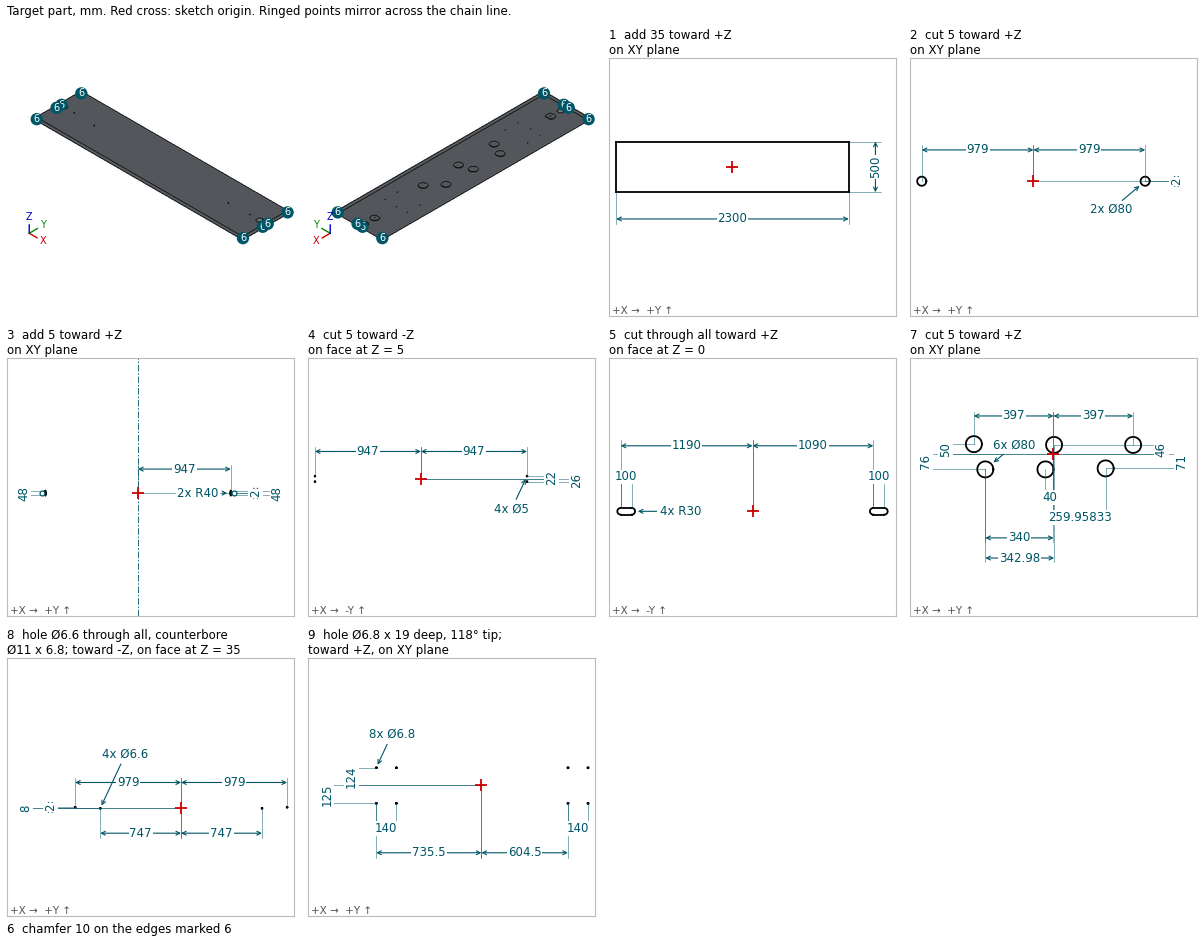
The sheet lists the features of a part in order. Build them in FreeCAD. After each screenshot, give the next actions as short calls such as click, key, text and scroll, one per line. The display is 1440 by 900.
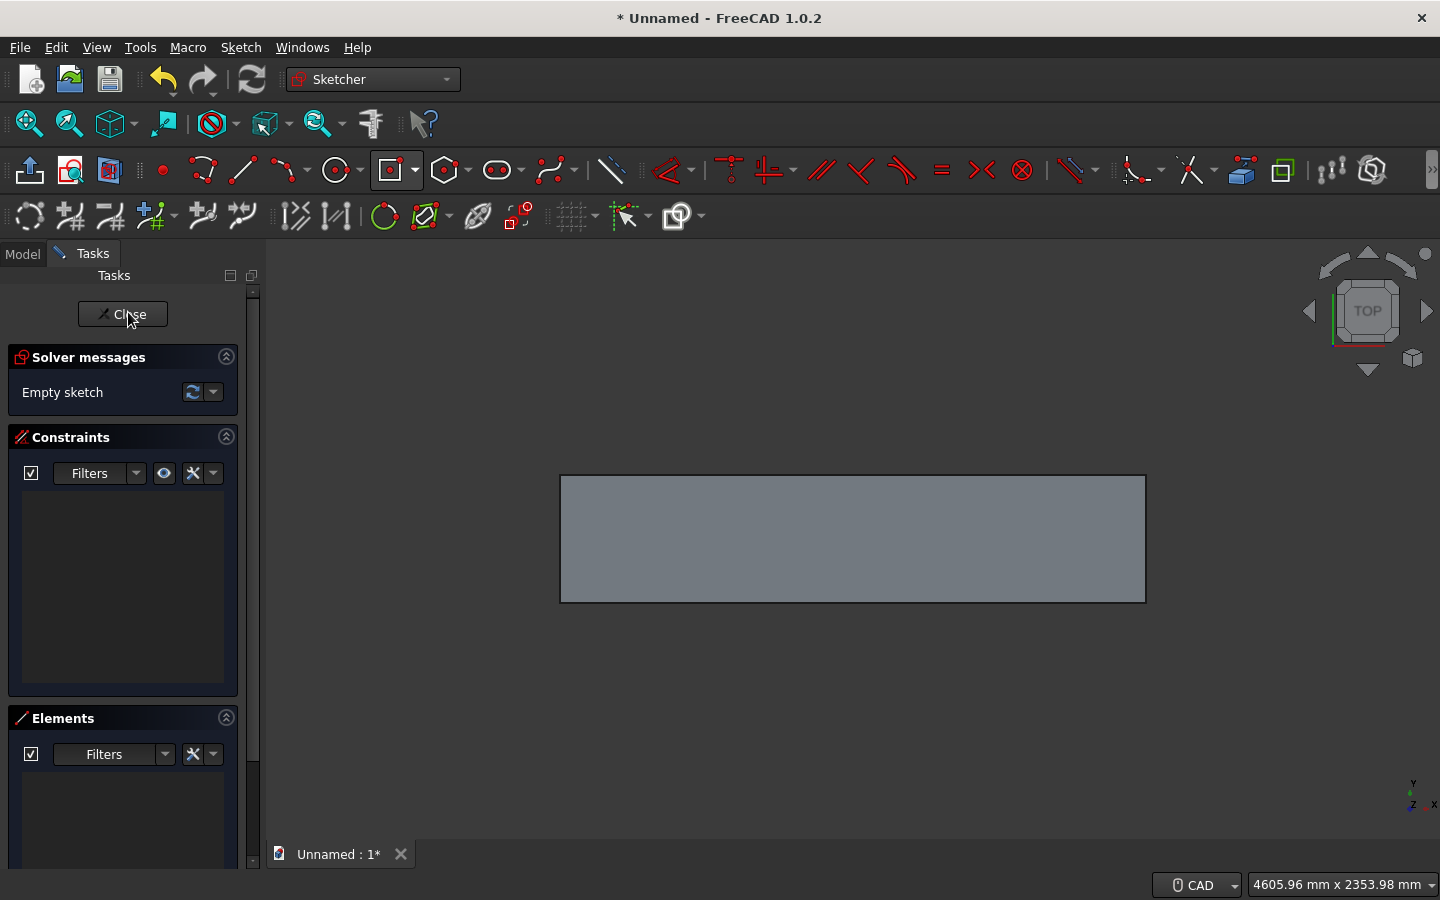
key(q)
key(s)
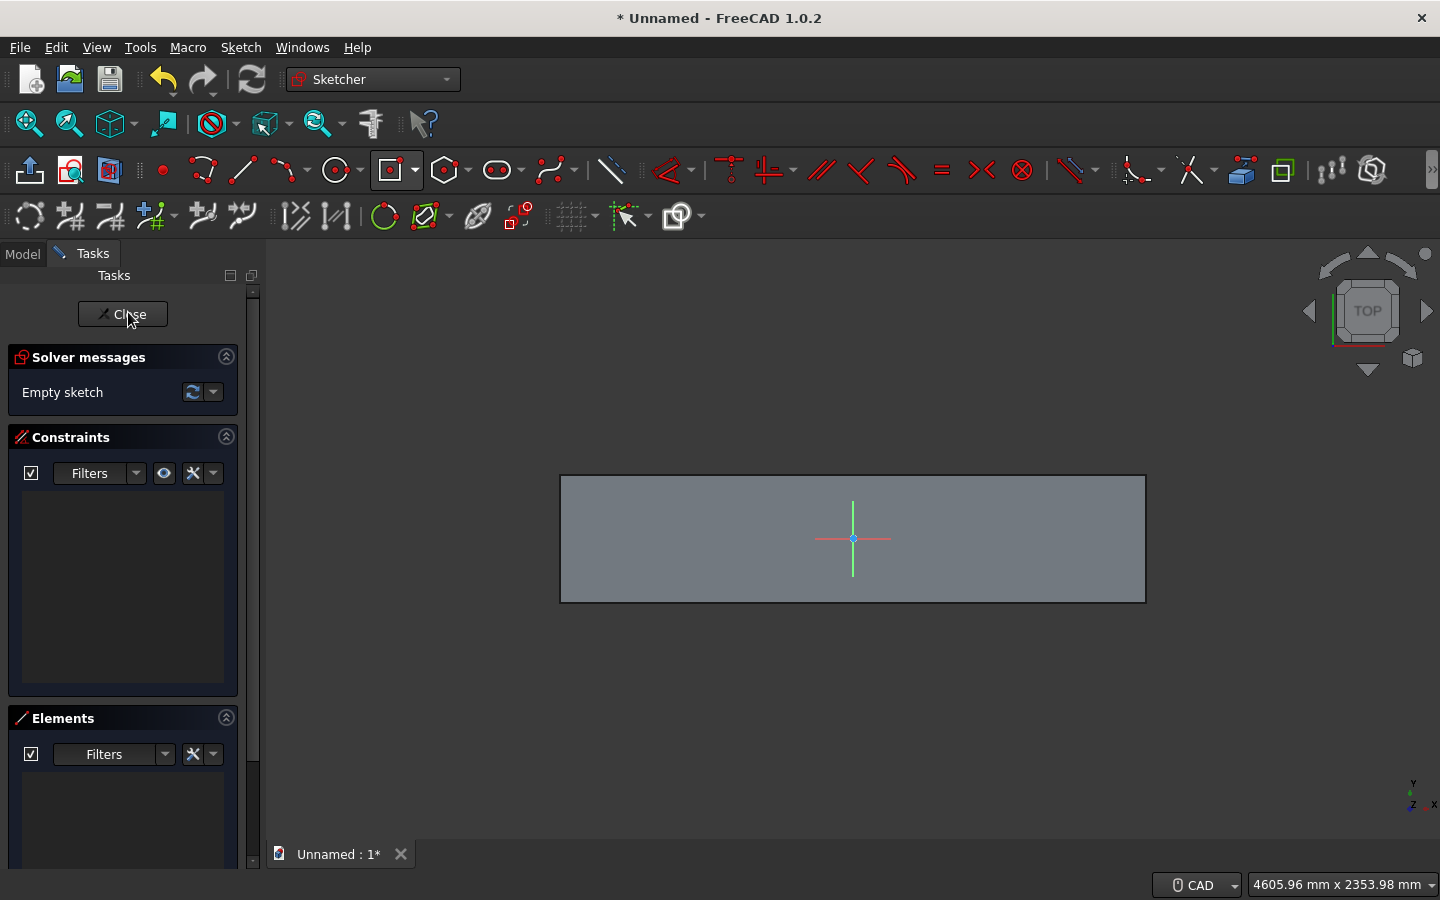
click(336, 170)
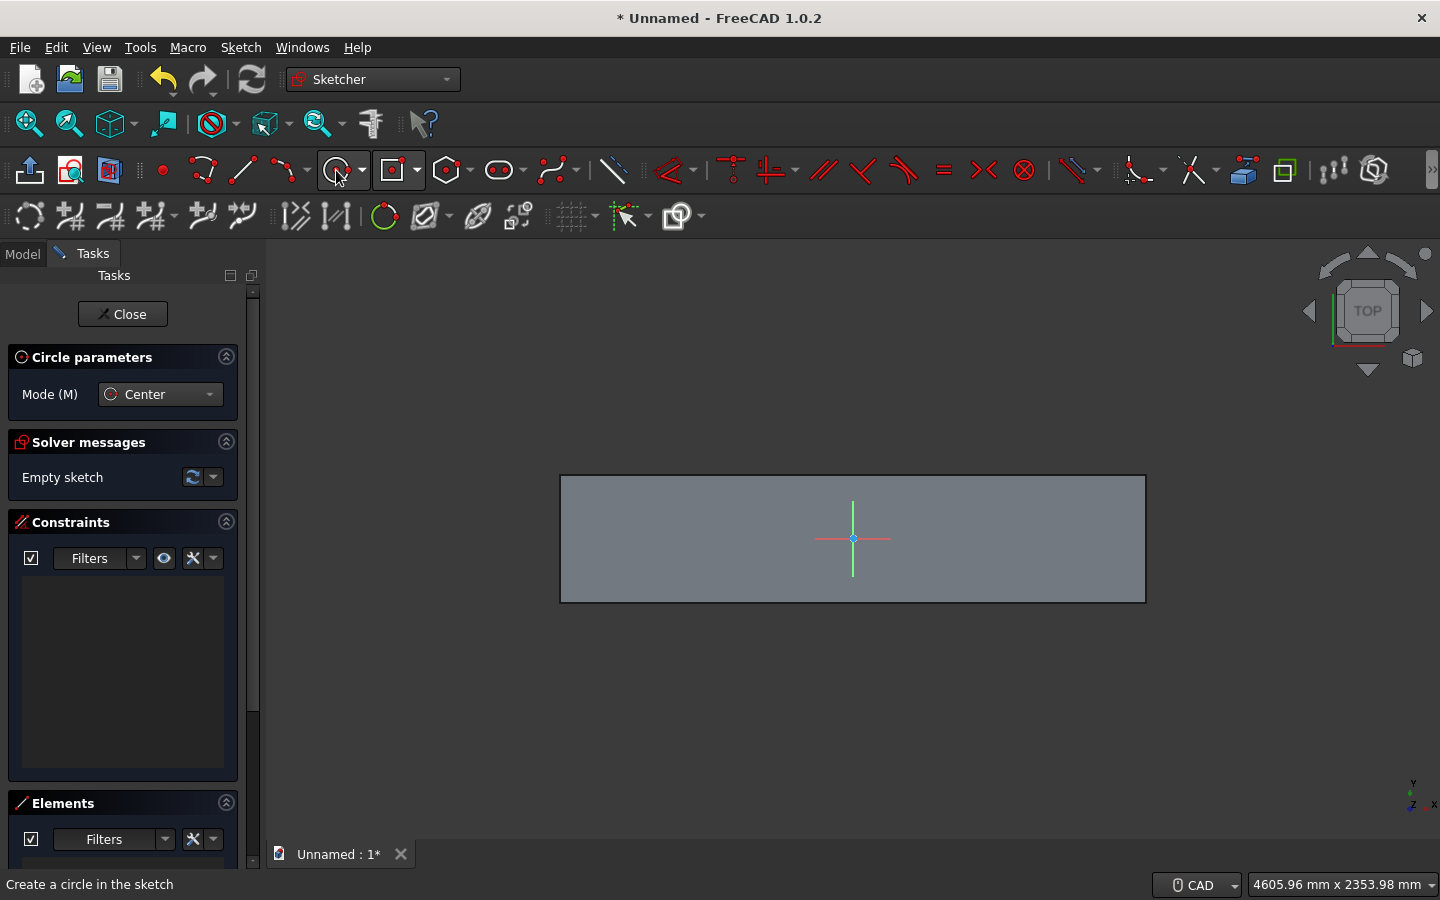
scroll(1103, 538, up, 18)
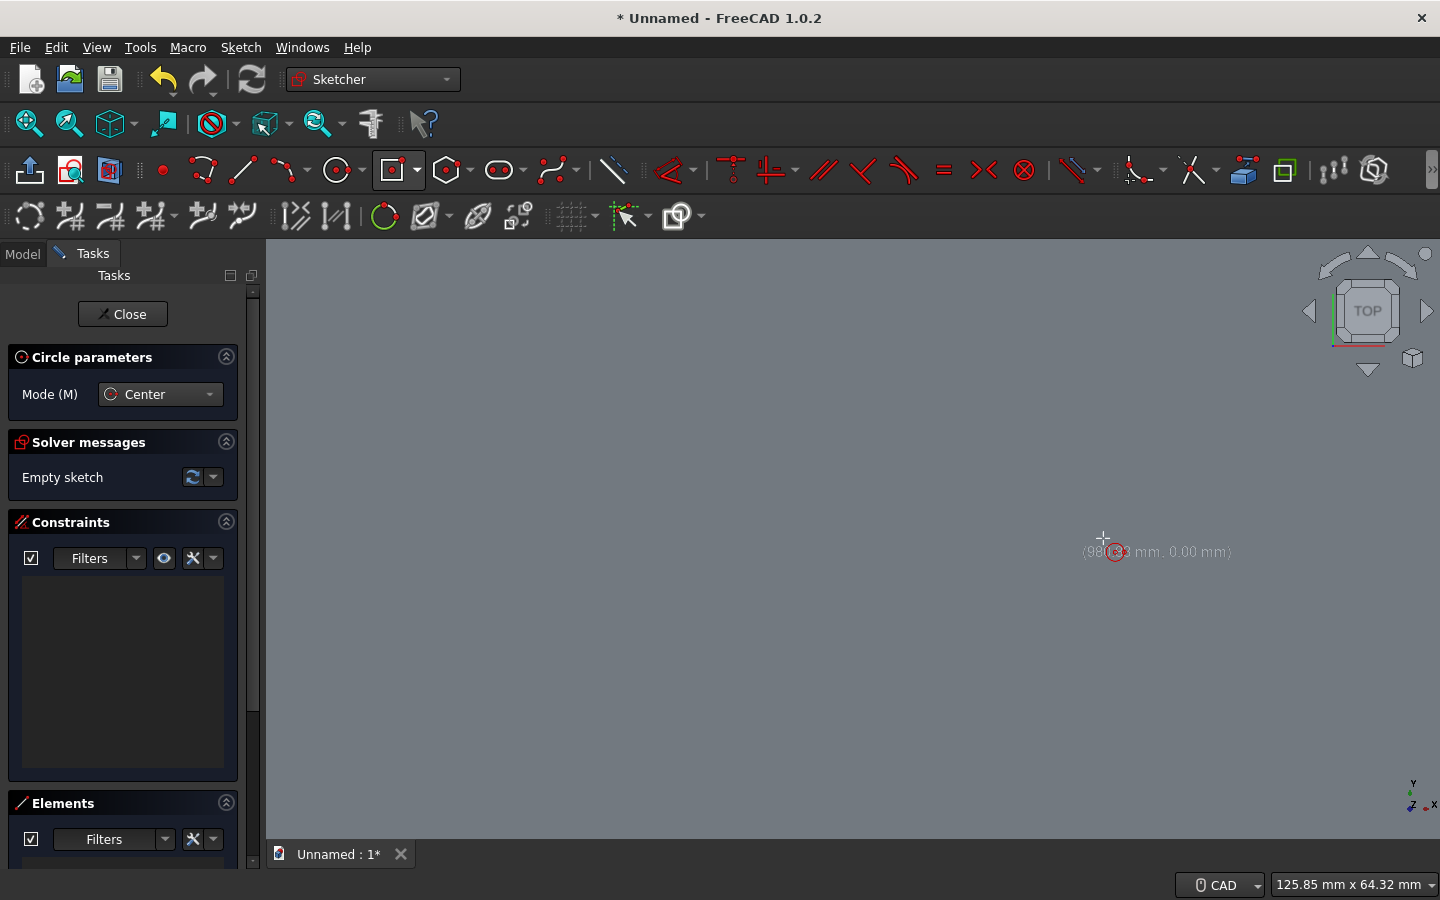
click(1061, 538)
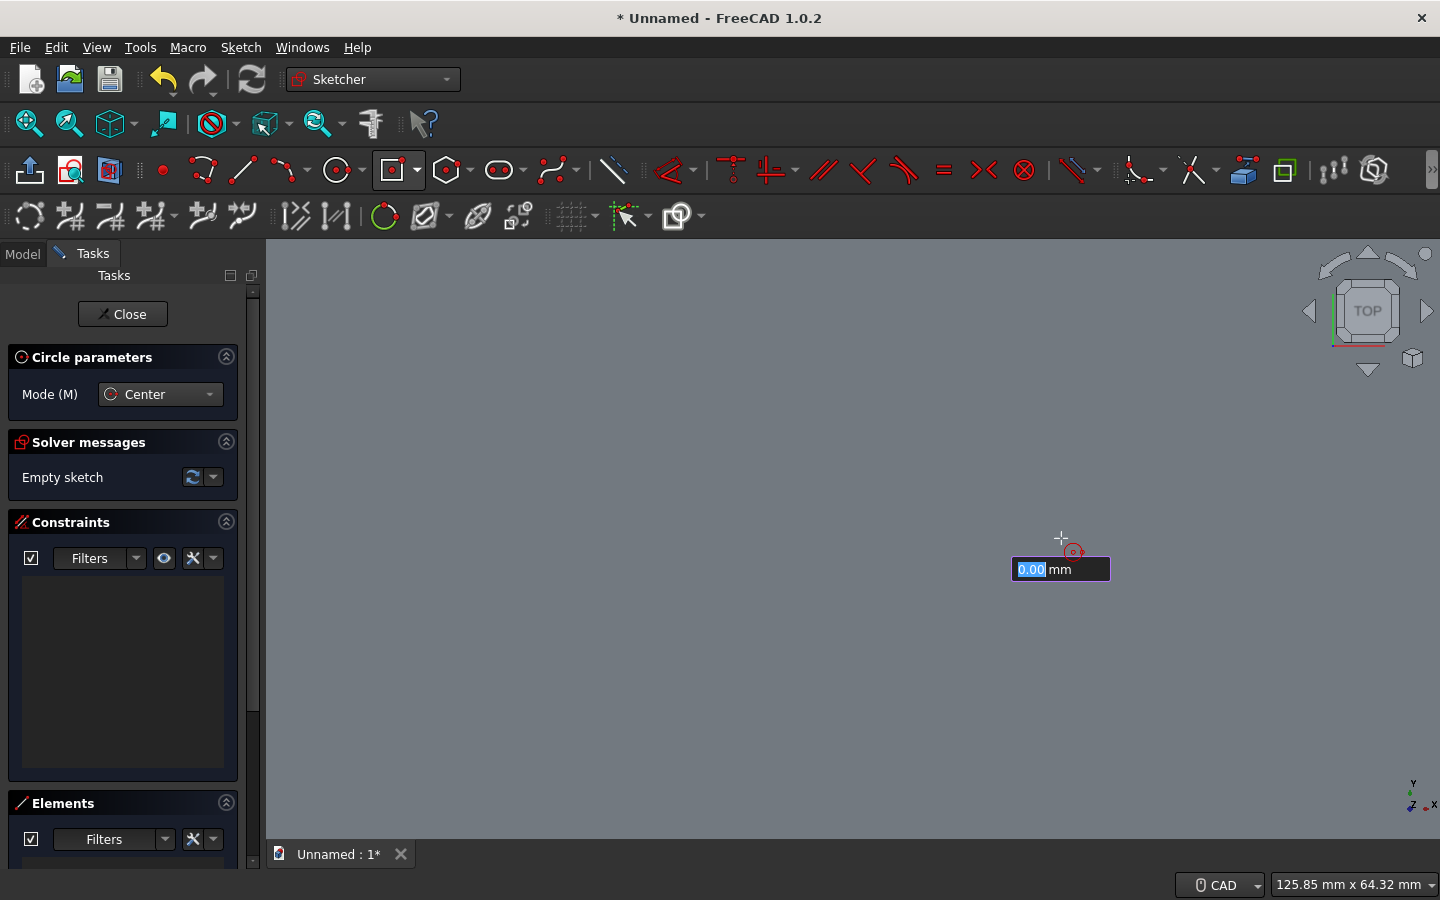
scroll(1161, 539, down, 16)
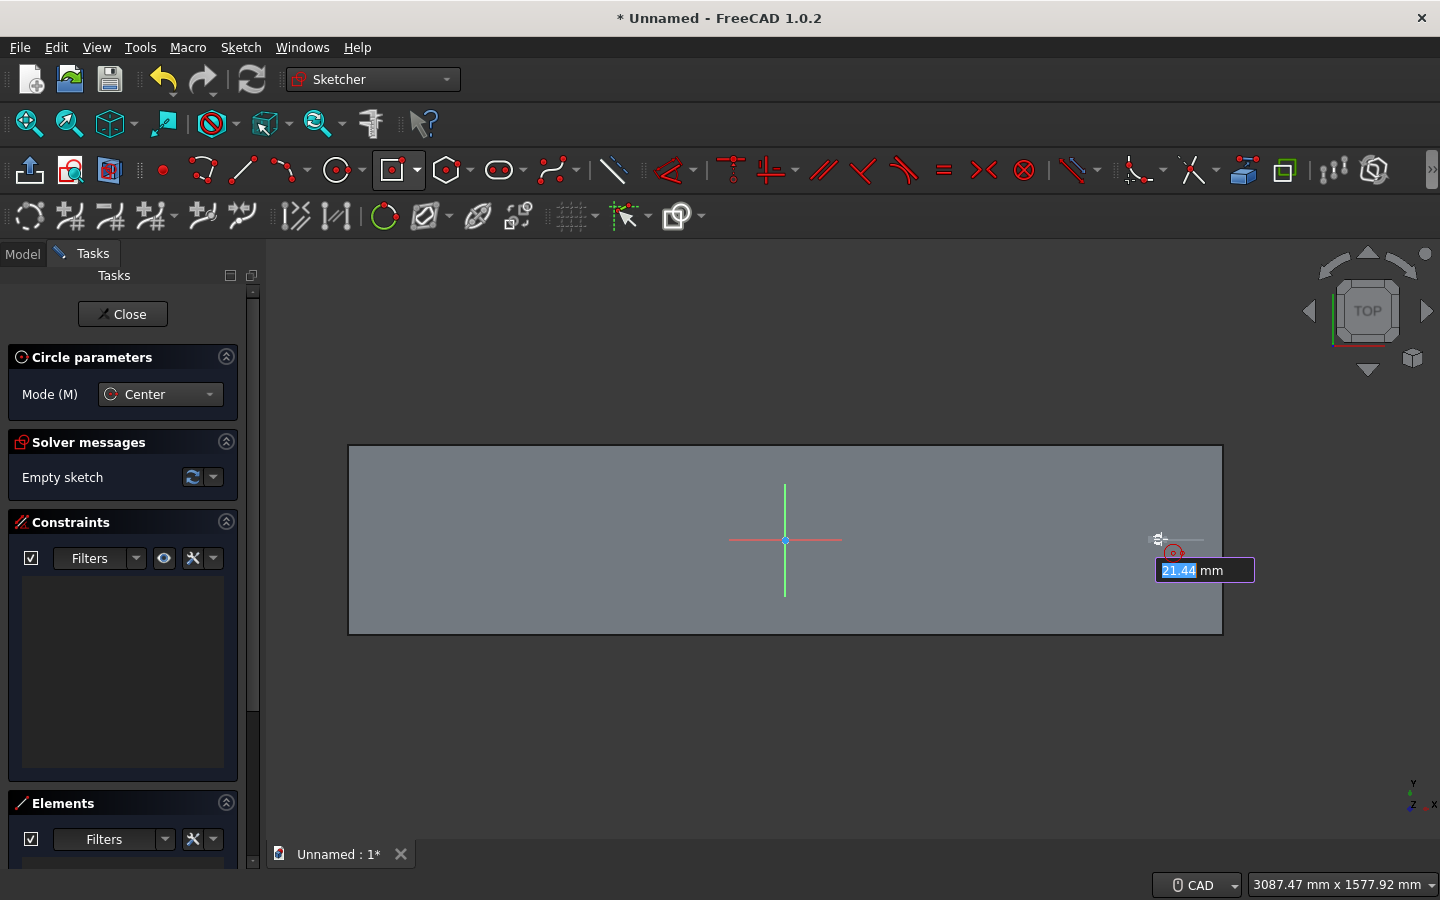
scroll(1168, 529, up, 2)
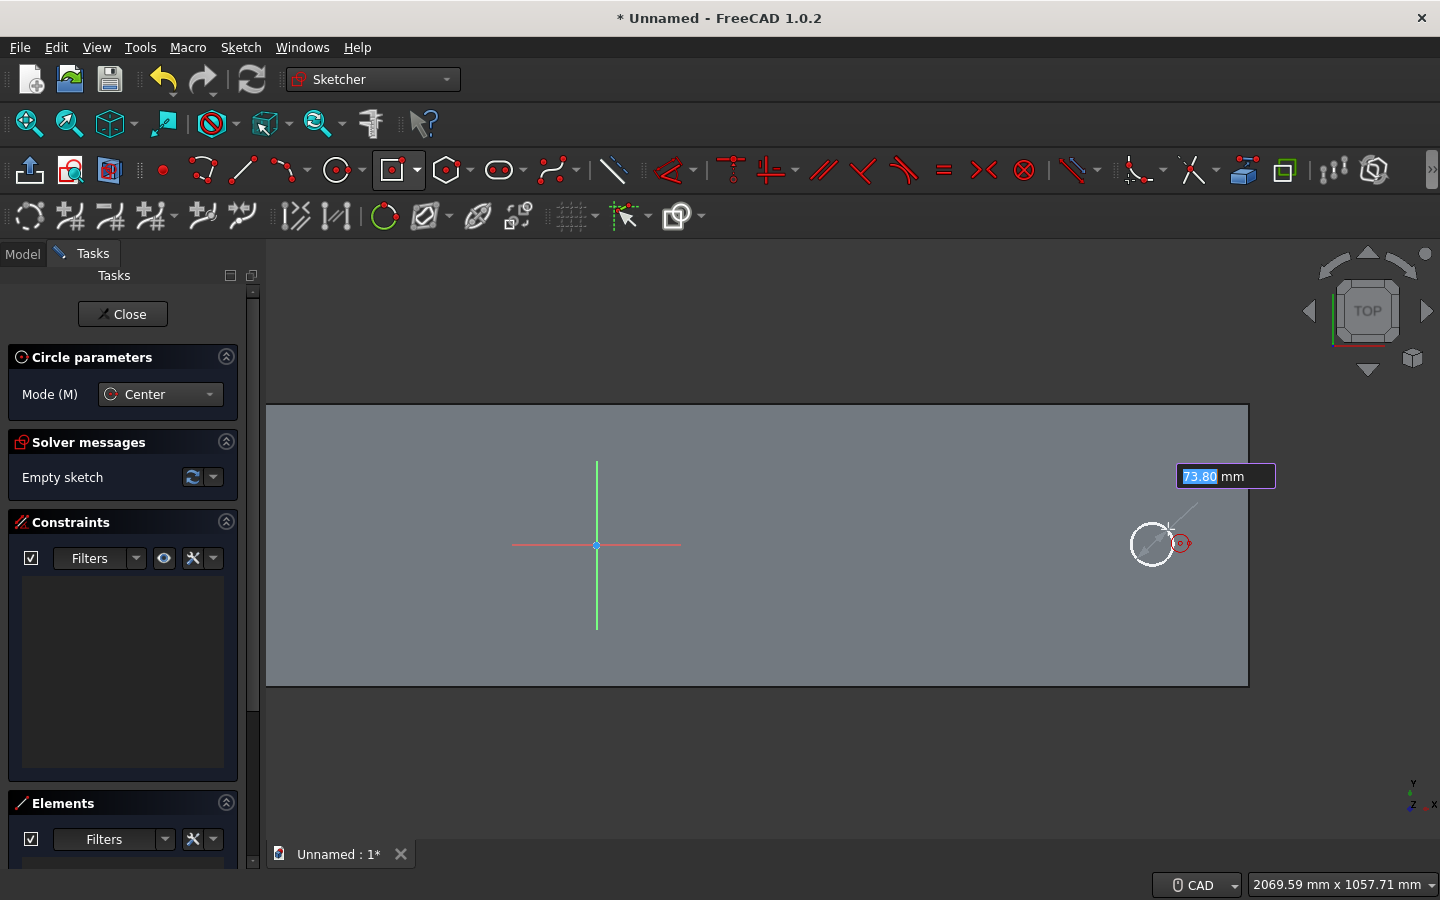
click(1168, 528)